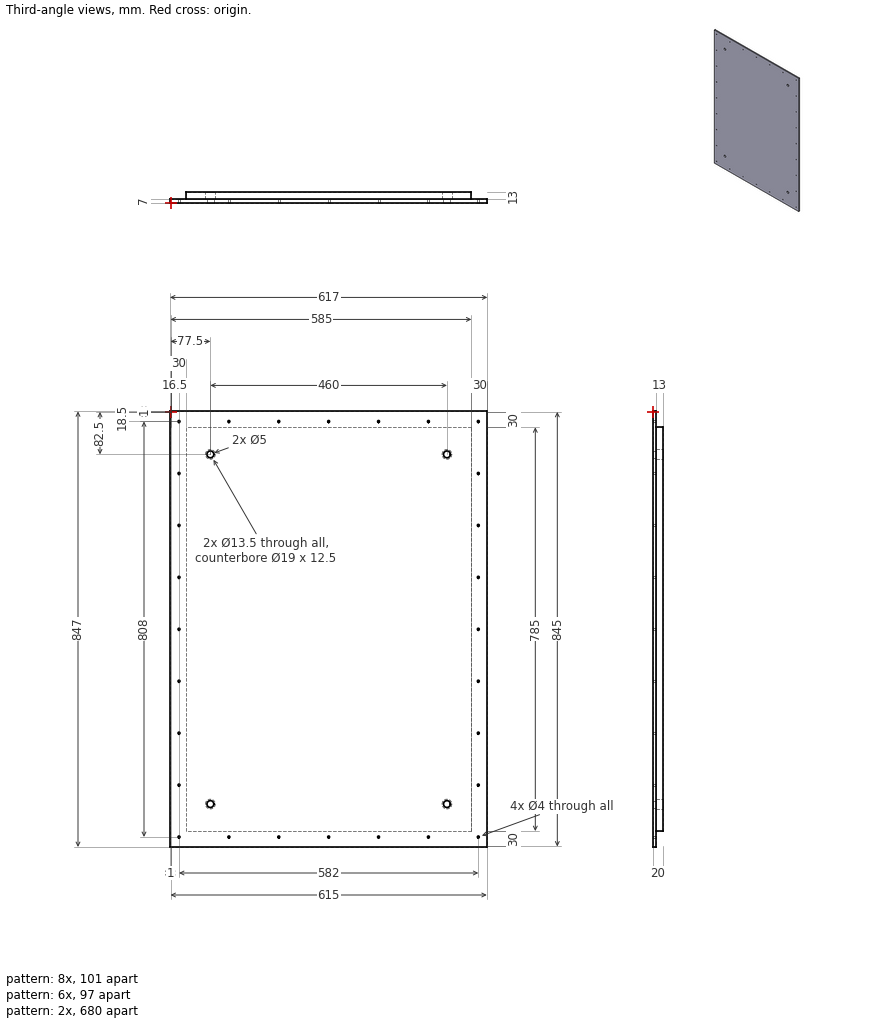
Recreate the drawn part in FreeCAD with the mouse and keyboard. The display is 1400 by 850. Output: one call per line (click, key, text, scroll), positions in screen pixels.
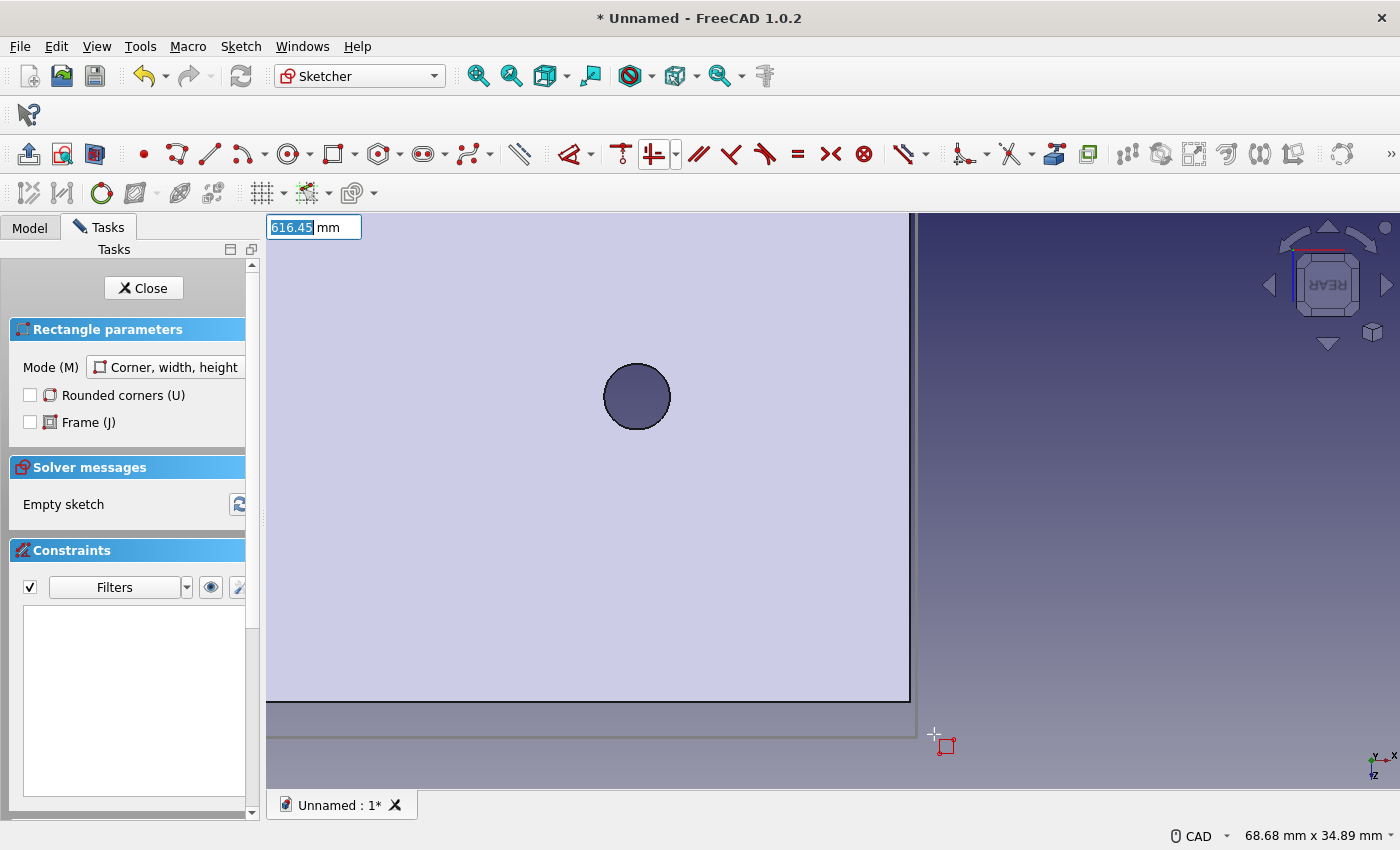
click(926, 719)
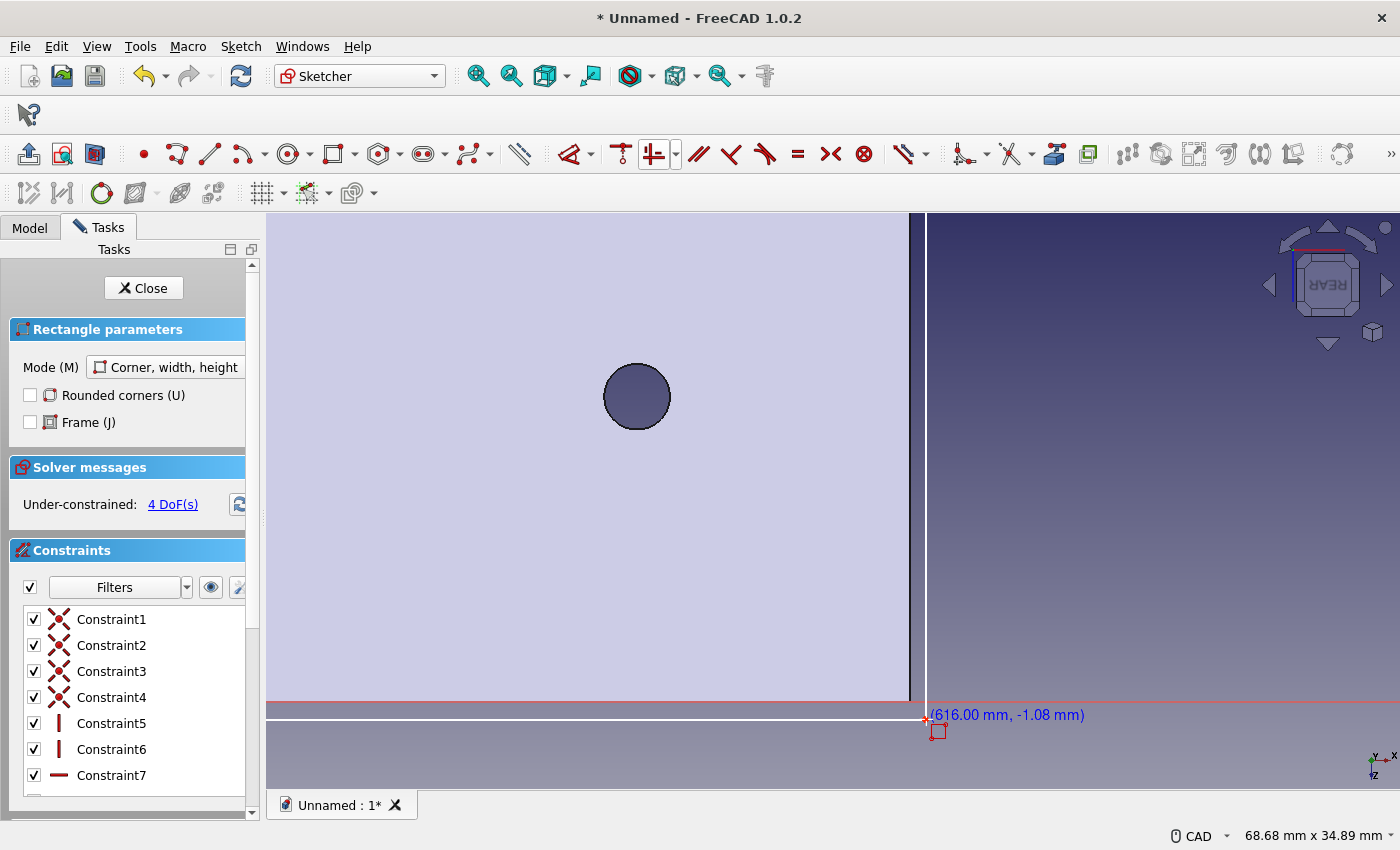
scroll(935, 735, down, 17)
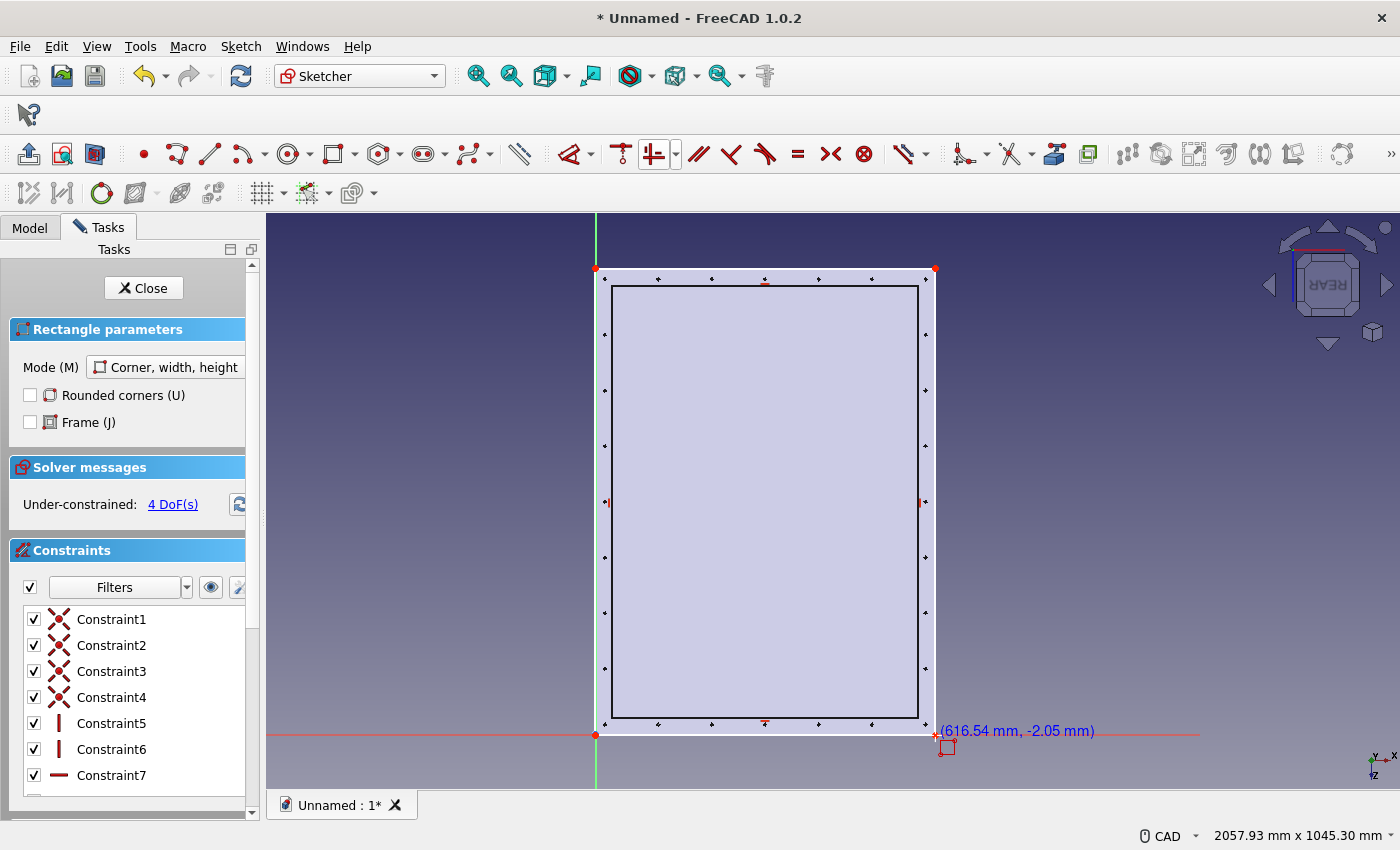
scroll(596, 735, up, 17)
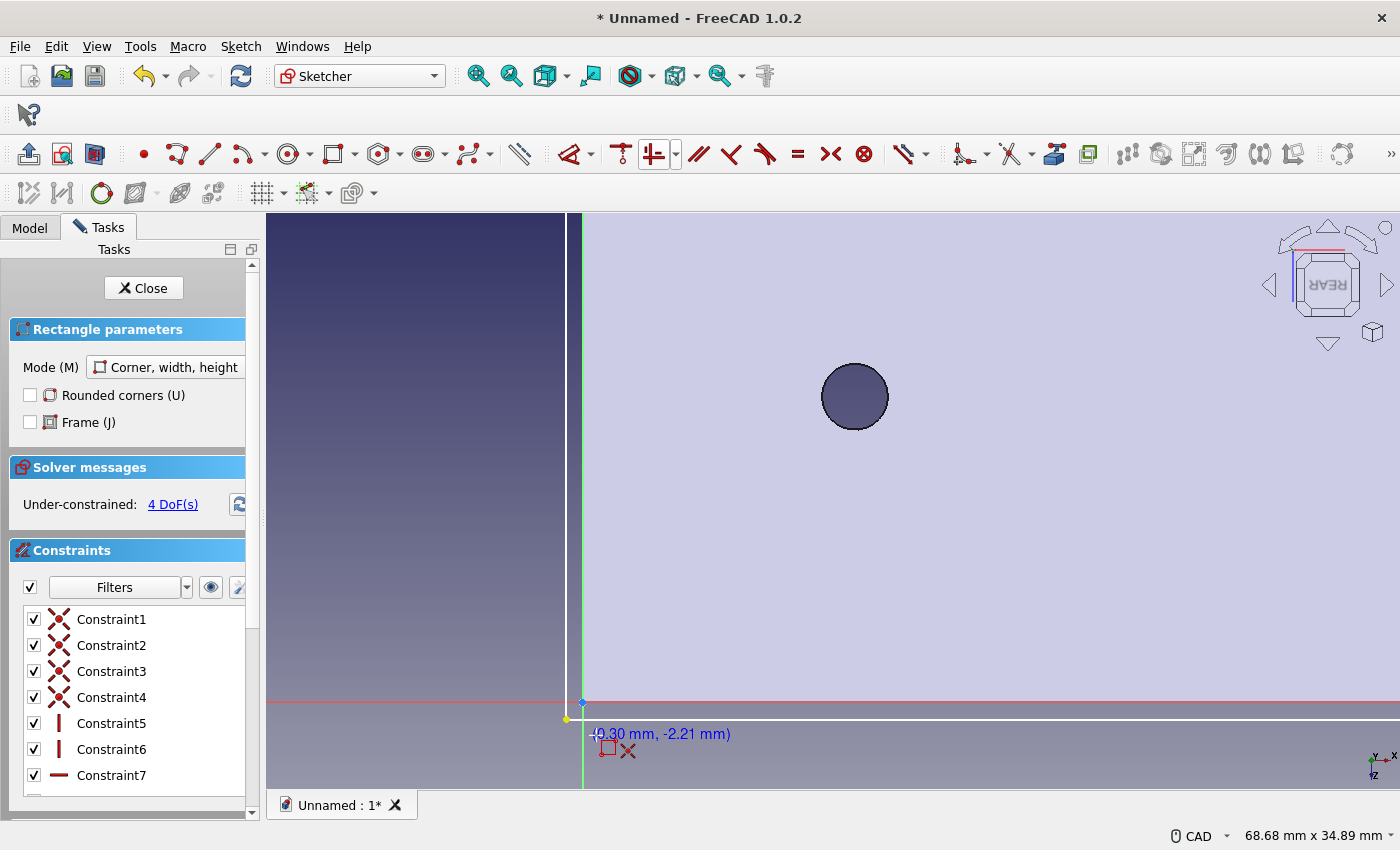
click(583, 702)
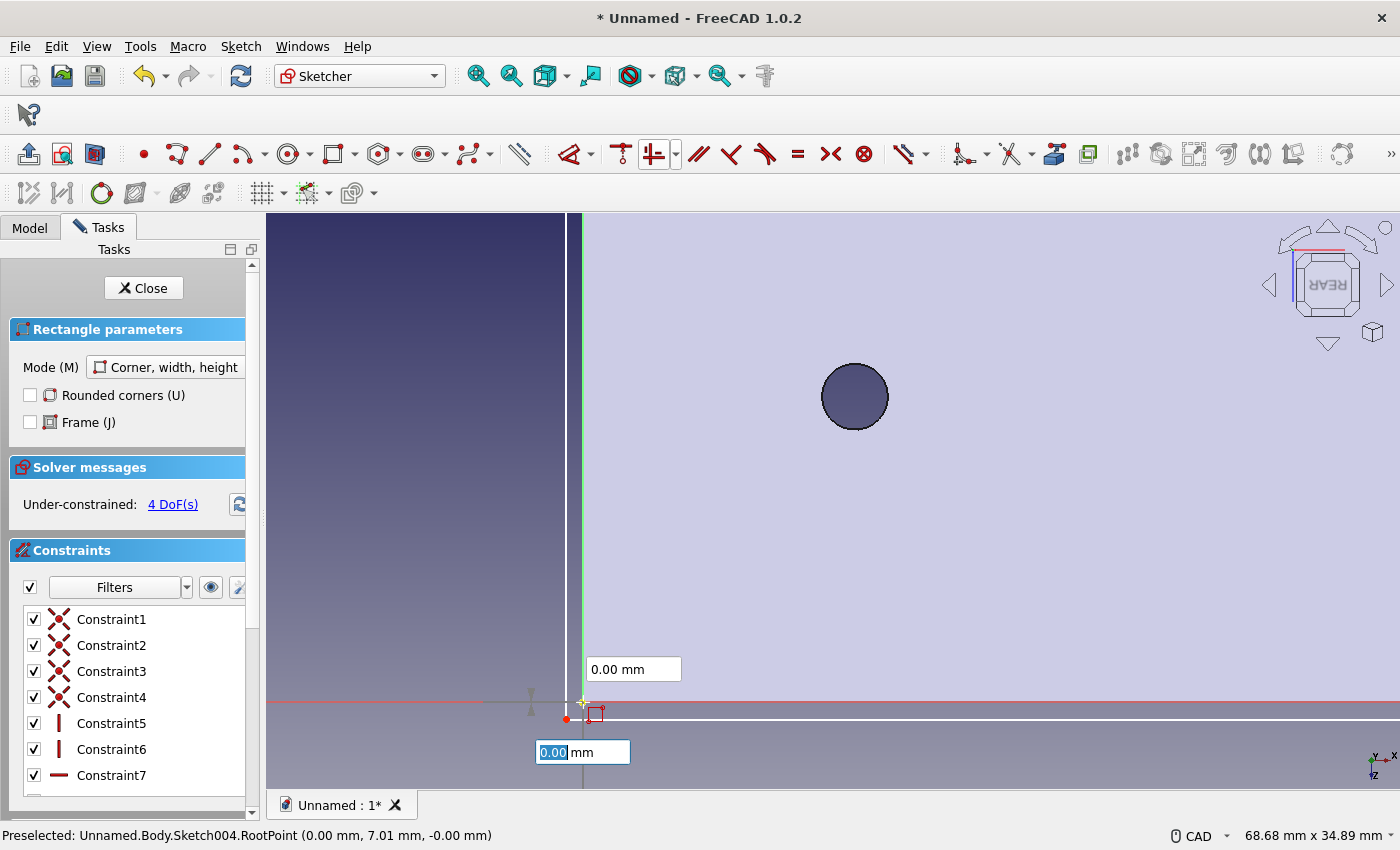
scroll(595, 735, down, 17)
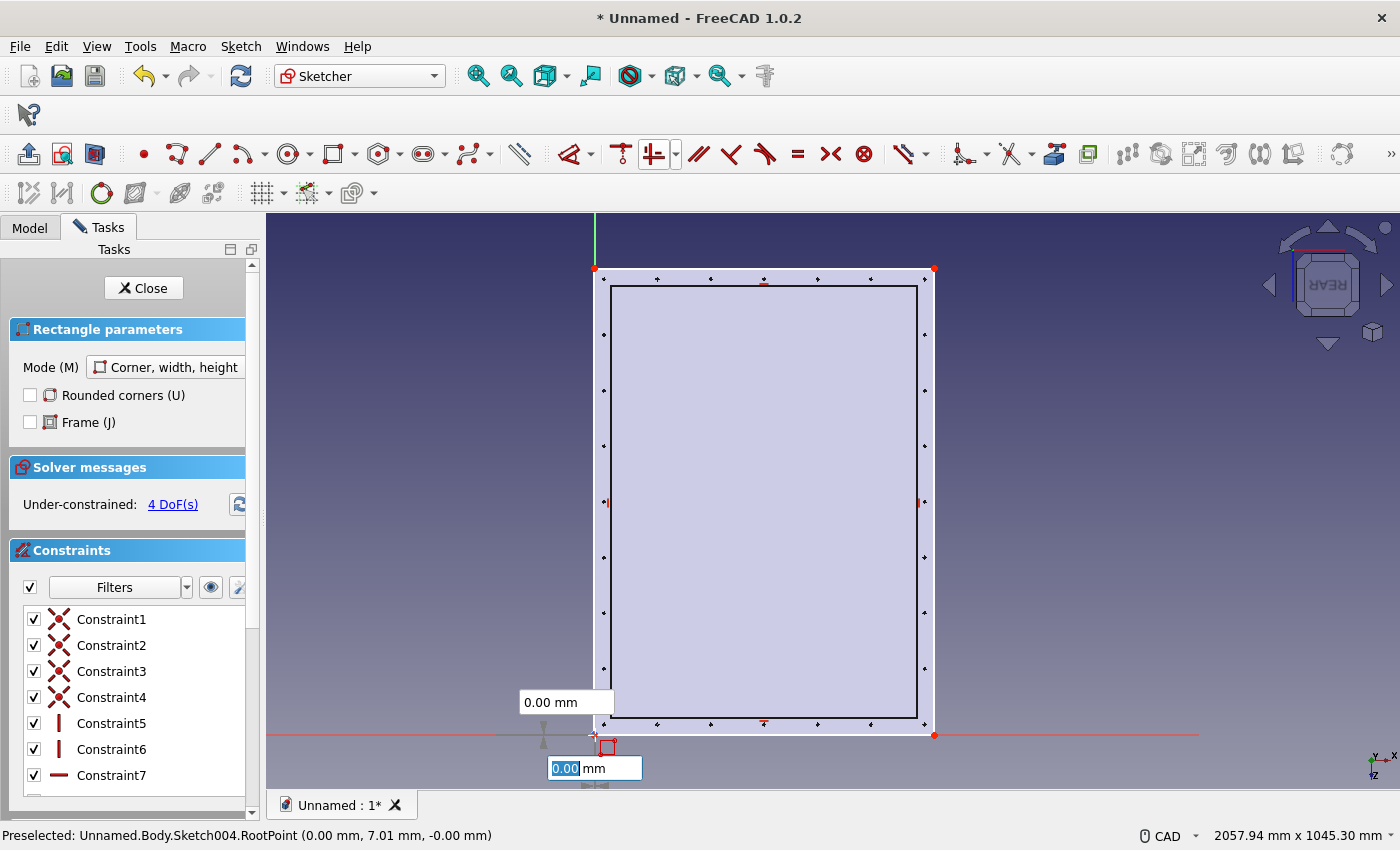
scroll(934, 269, up, 17)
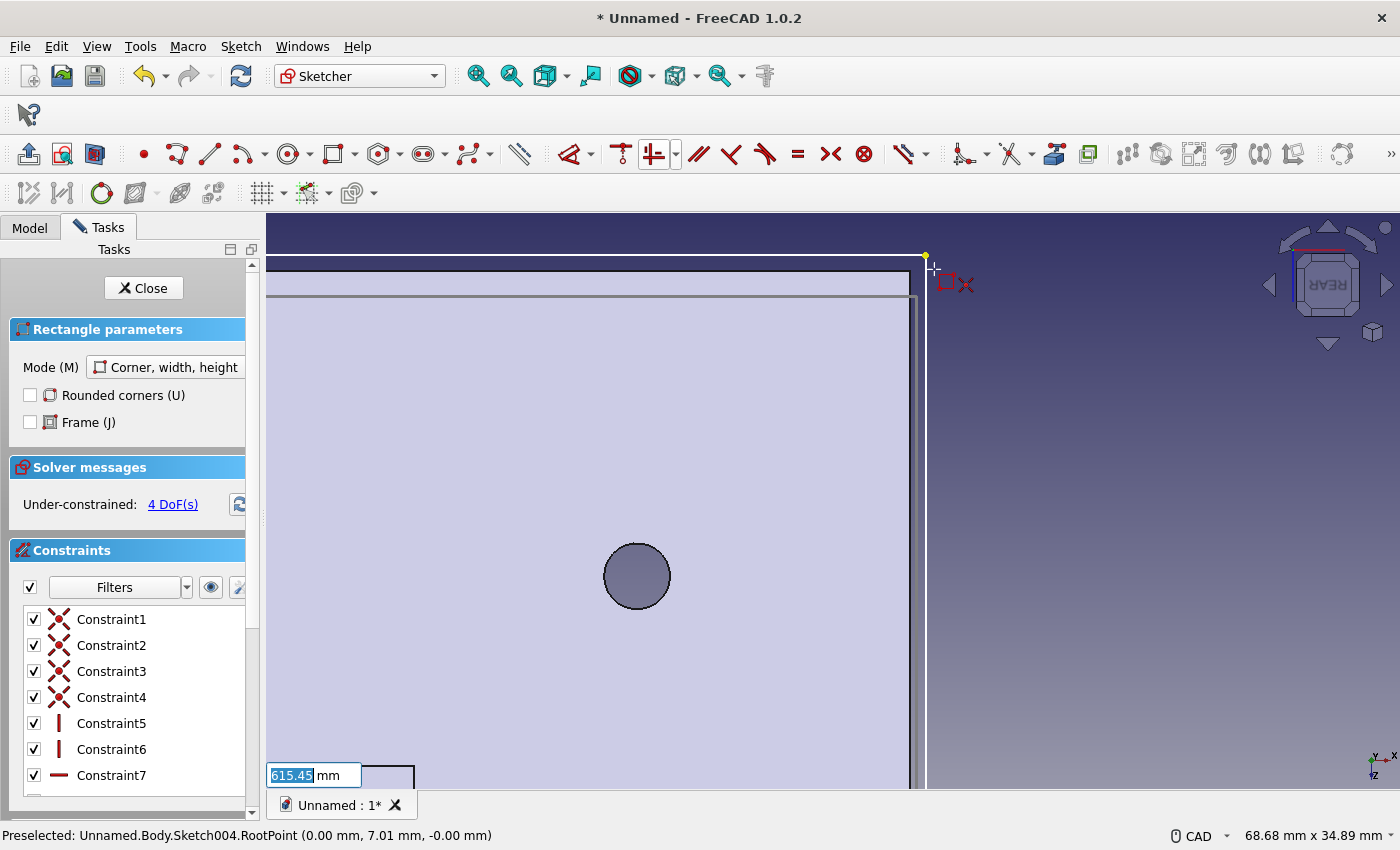
click(910, 271)
key(Escape)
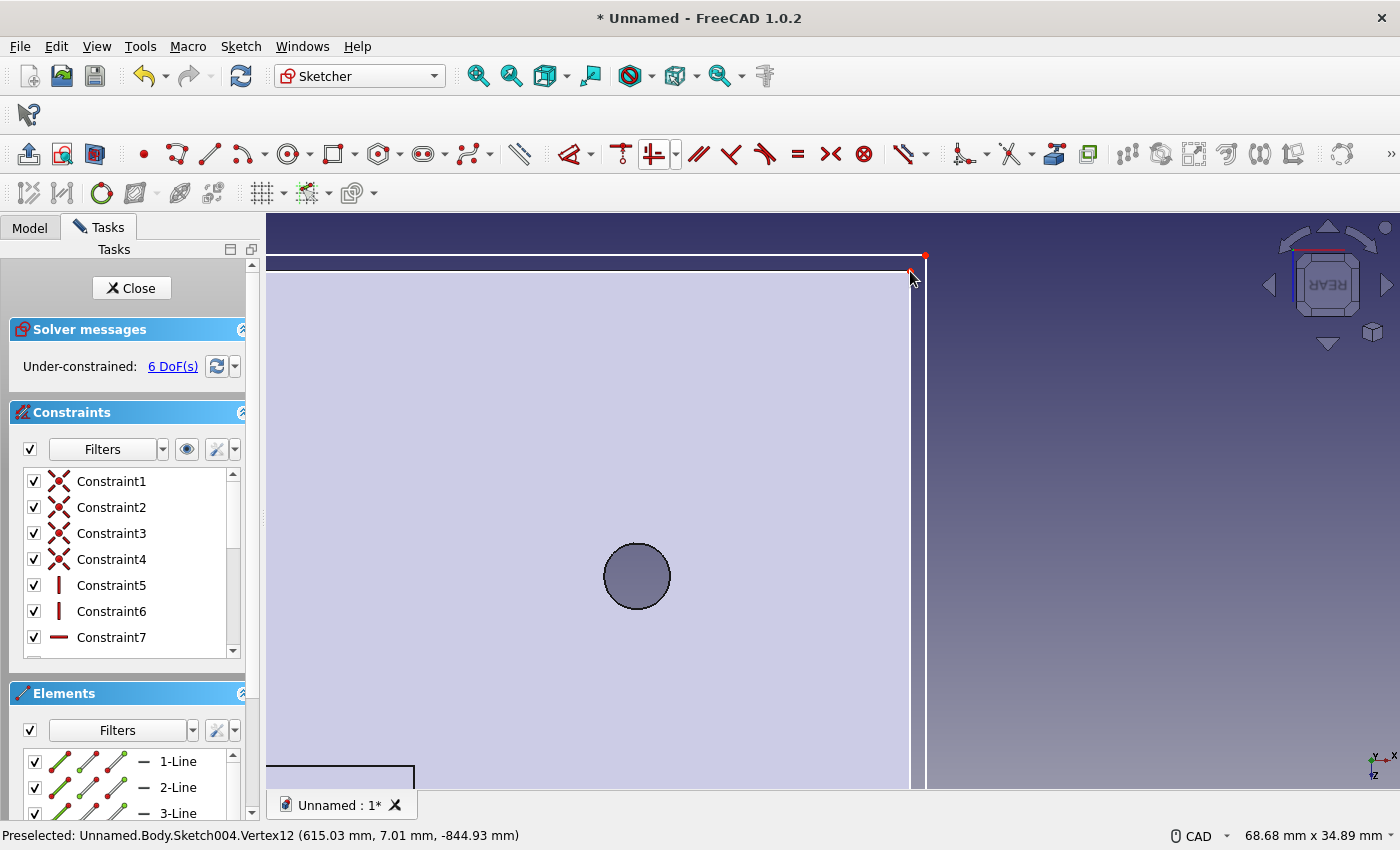
click(568, 154)